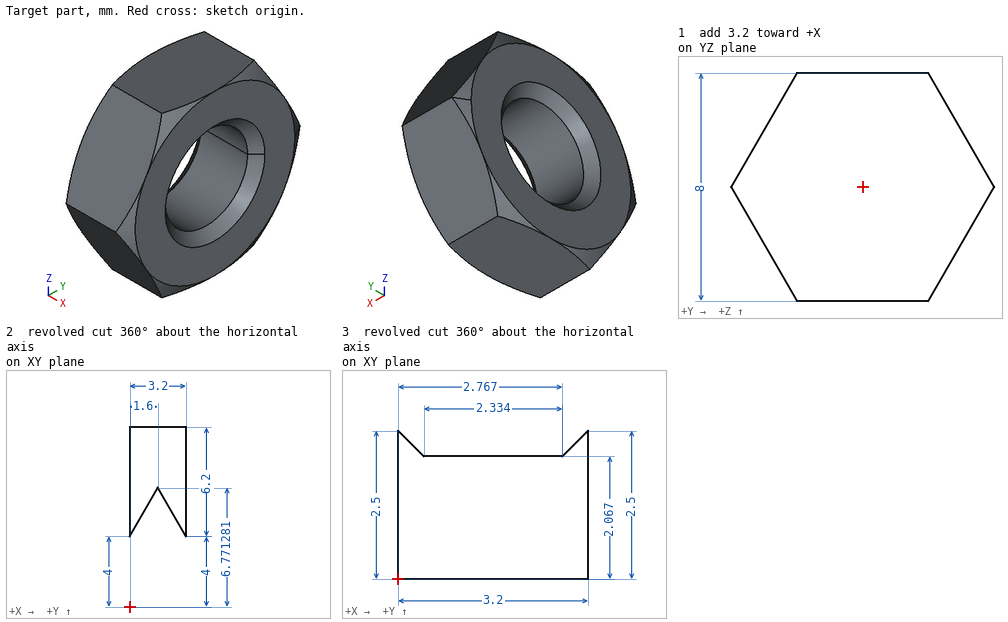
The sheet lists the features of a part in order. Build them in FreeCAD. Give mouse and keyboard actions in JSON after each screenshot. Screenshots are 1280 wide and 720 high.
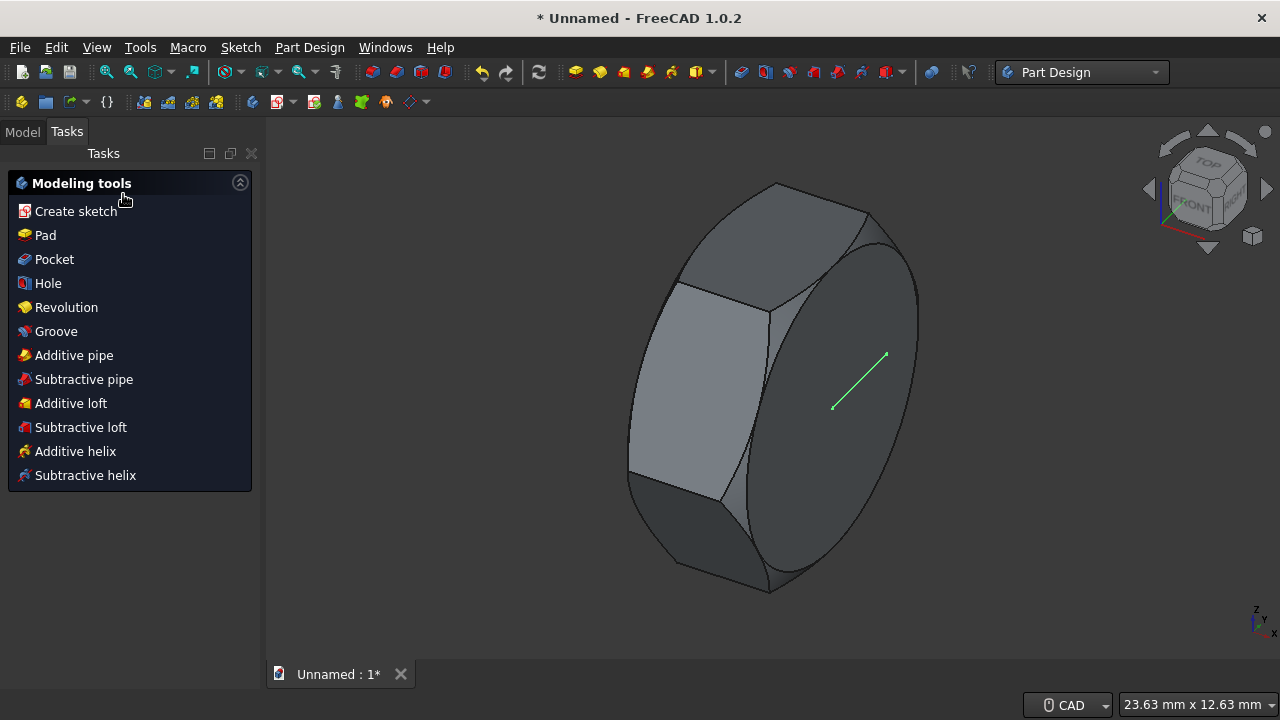
{"action": "left_click", "coordinate": [790, 72]}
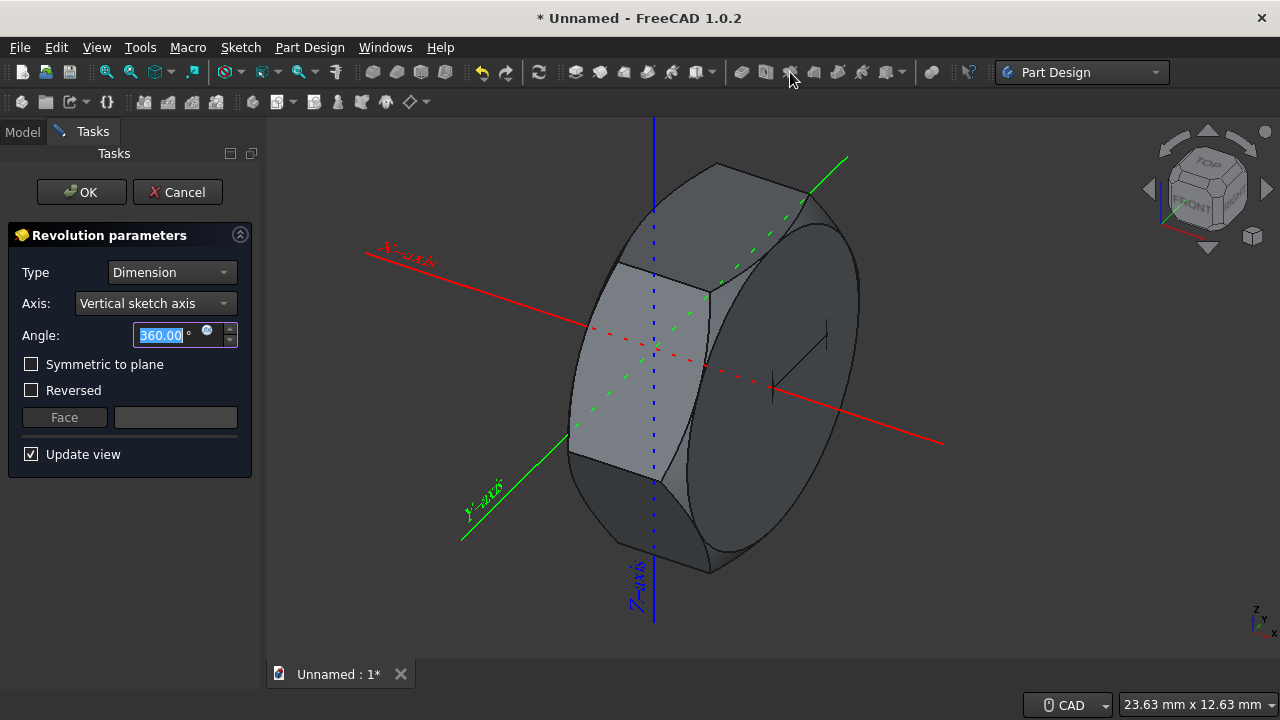
{"action": "left_click", "coordinate": [156, 304]}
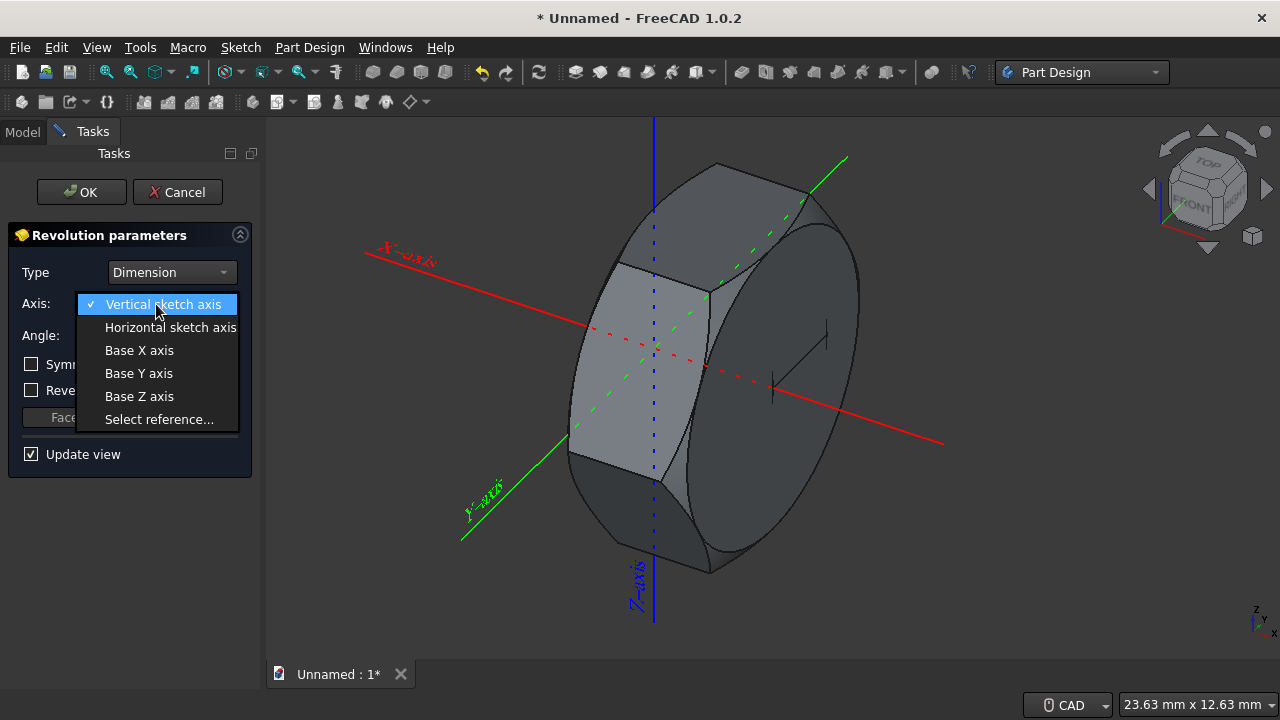
{"action": "left_click", "coordinate": [156, 328]}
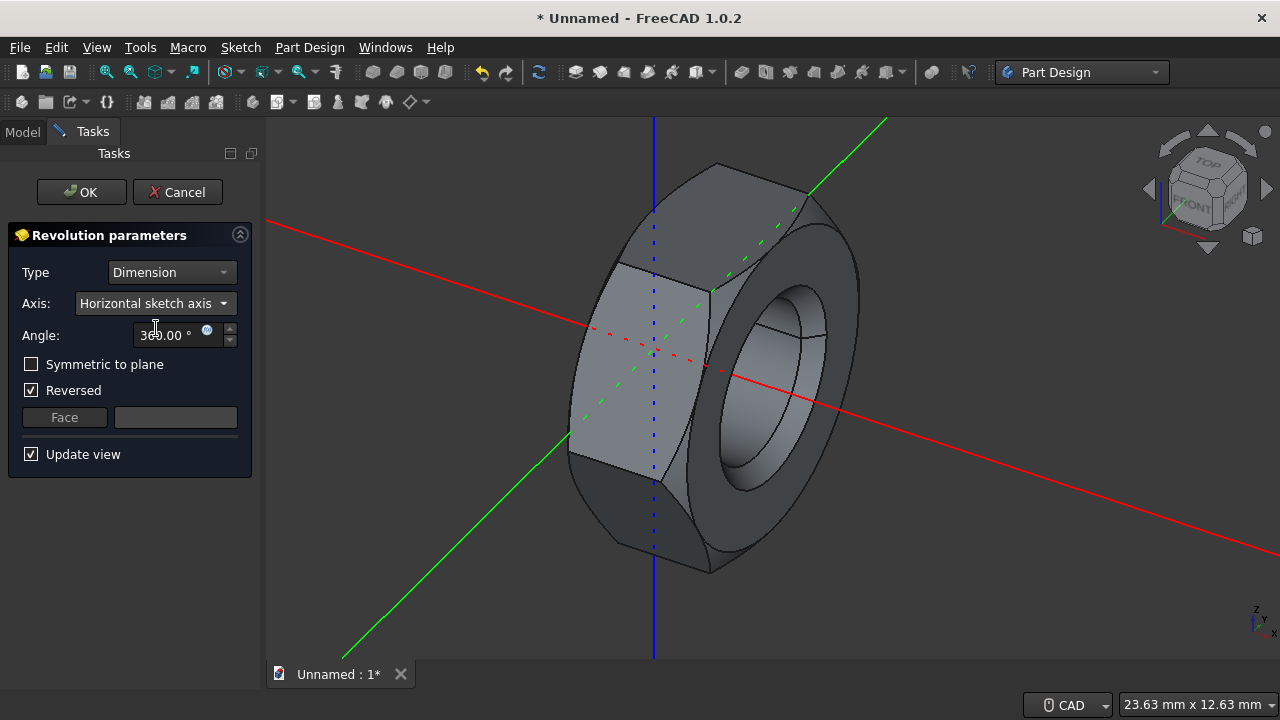
{"action": "left_click", "coordinate": [82, 192]}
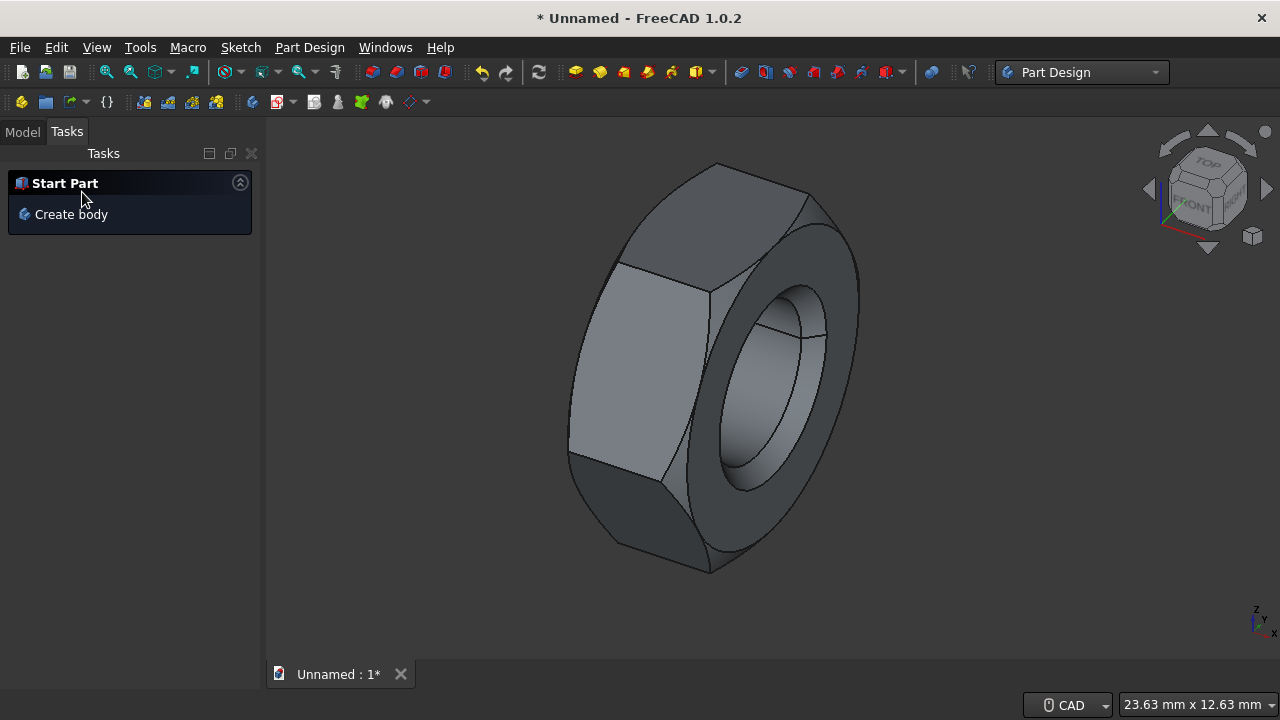
{"action": "key", "text": "0"}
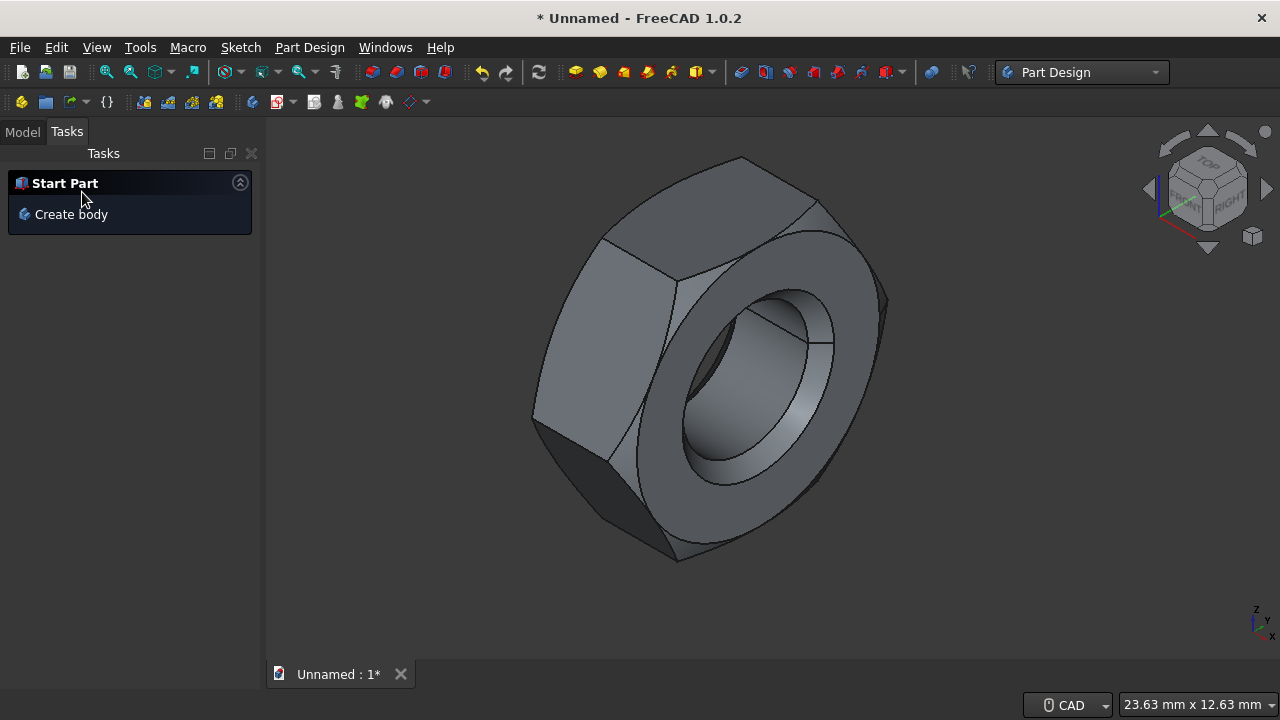
{"action": "key", "text": "v f"}